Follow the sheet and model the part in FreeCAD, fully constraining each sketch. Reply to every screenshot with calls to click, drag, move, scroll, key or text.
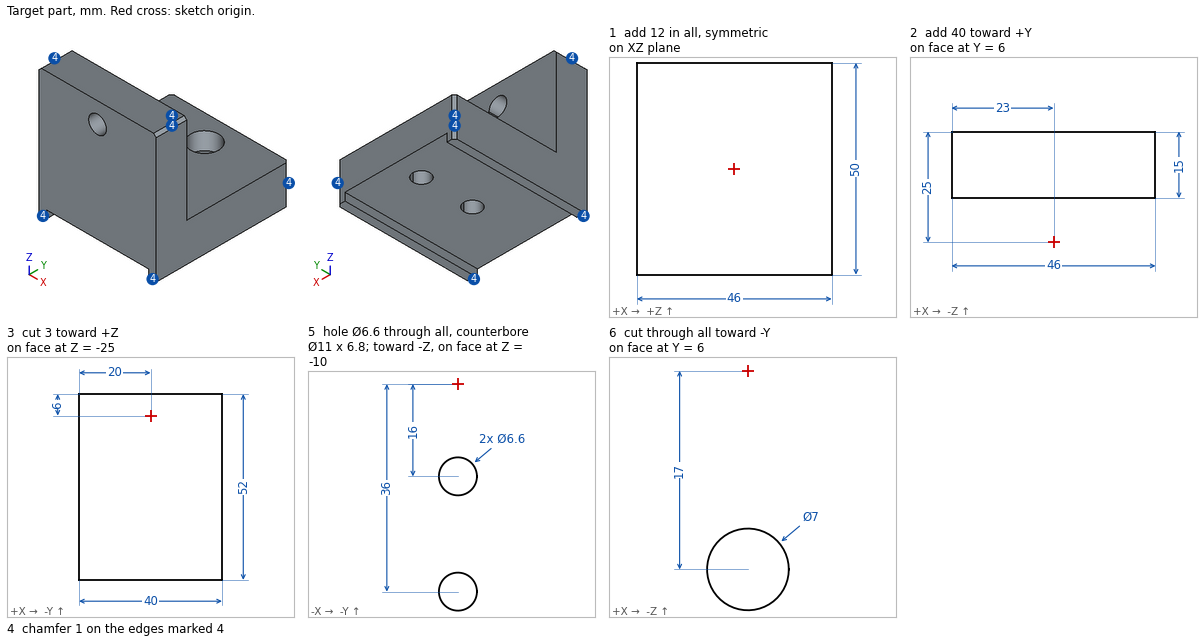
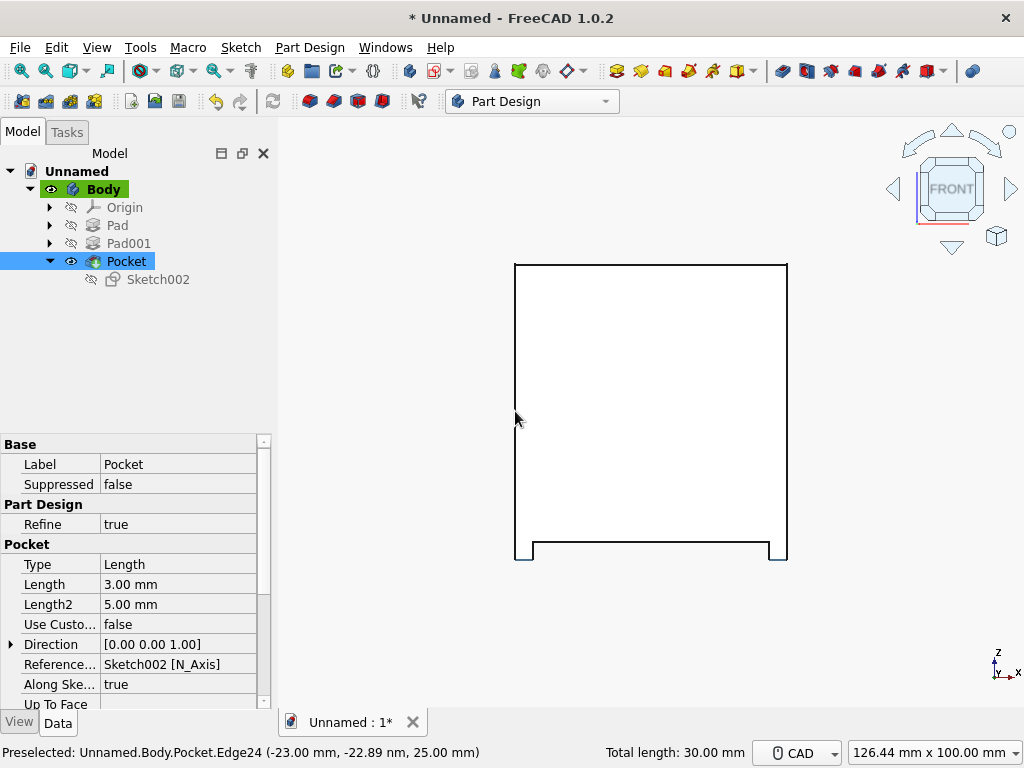
key(3)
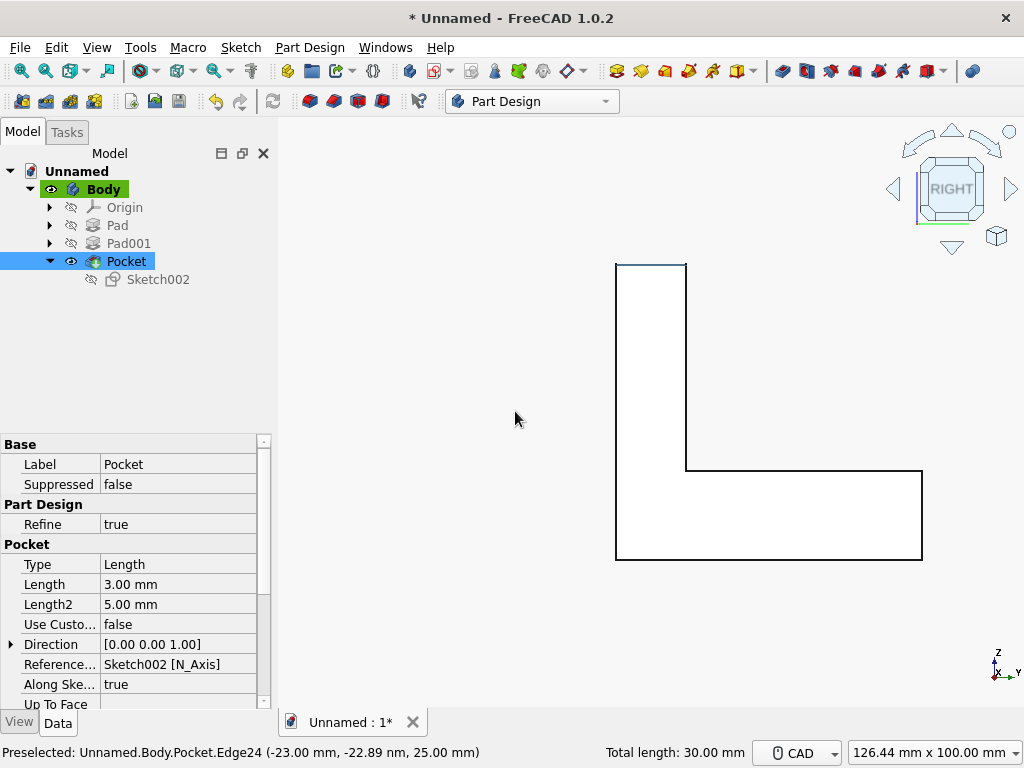
click(922, 514, ctrl)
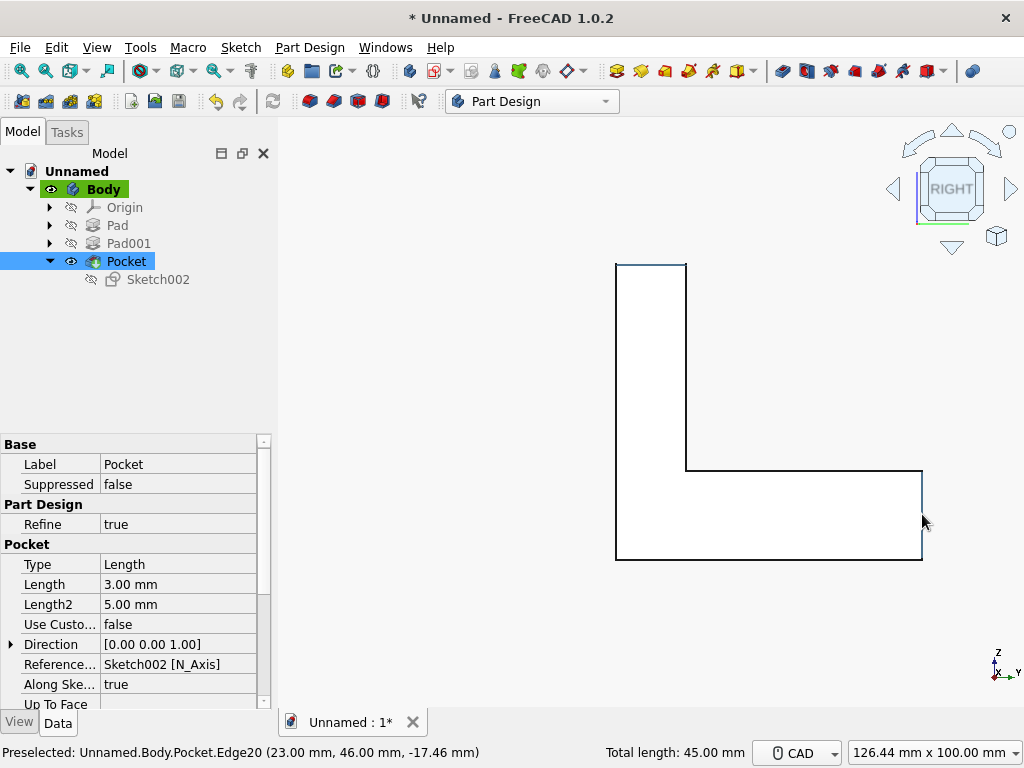
key(5)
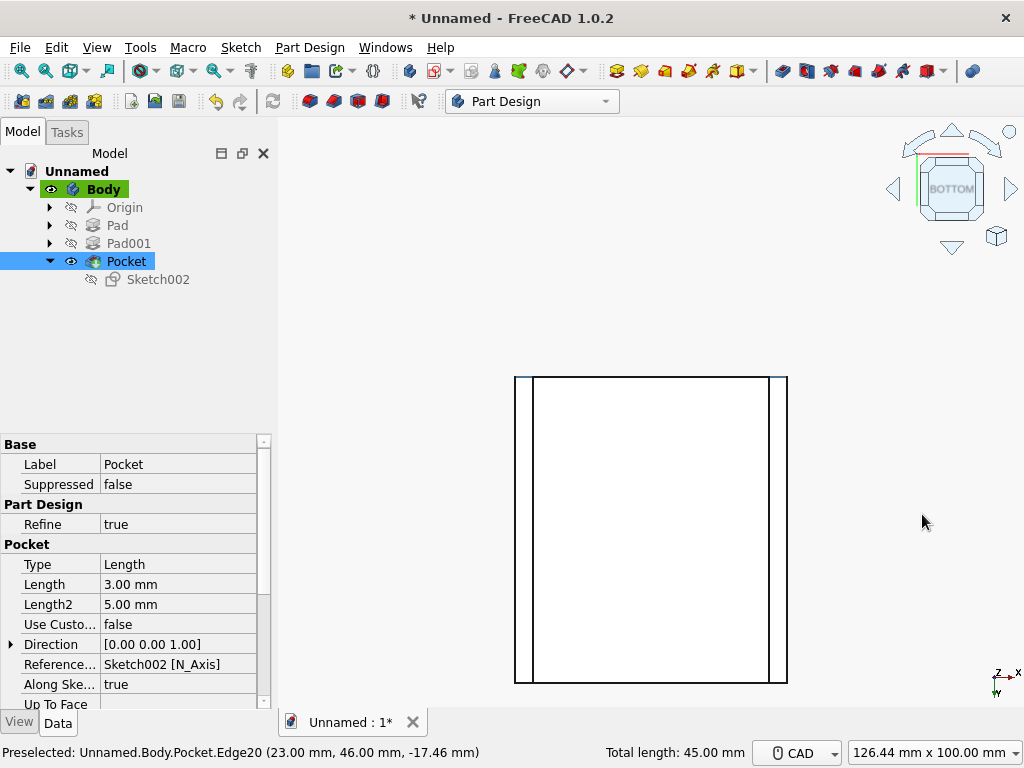
key(4)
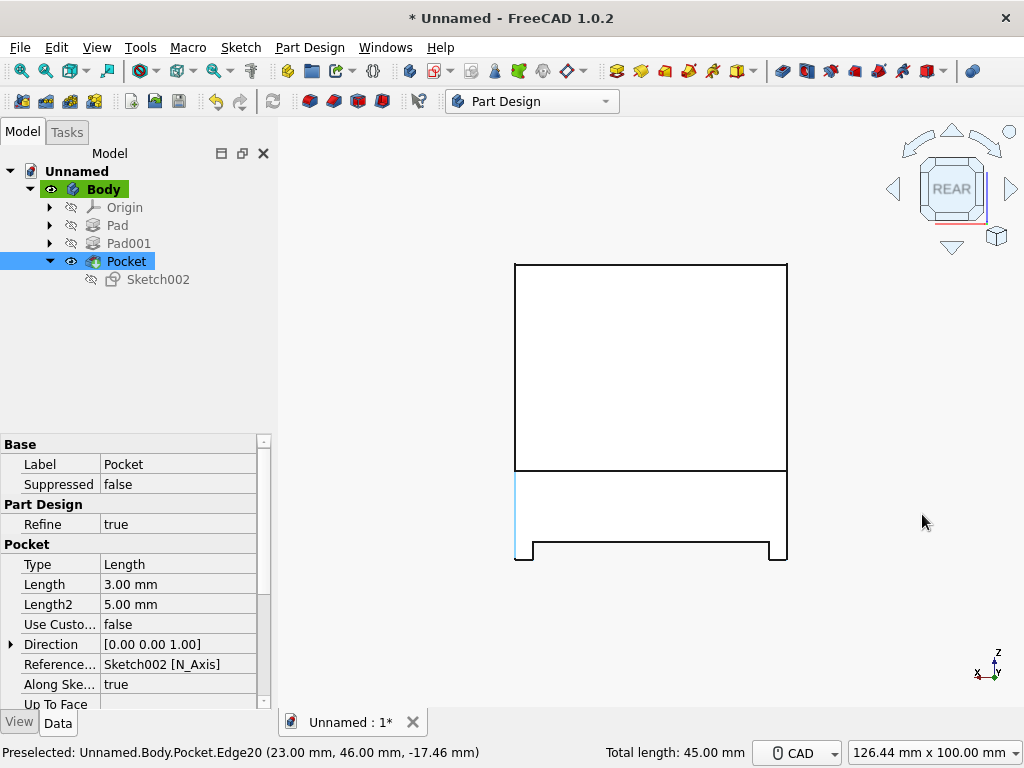
click(787, 514, ctrl)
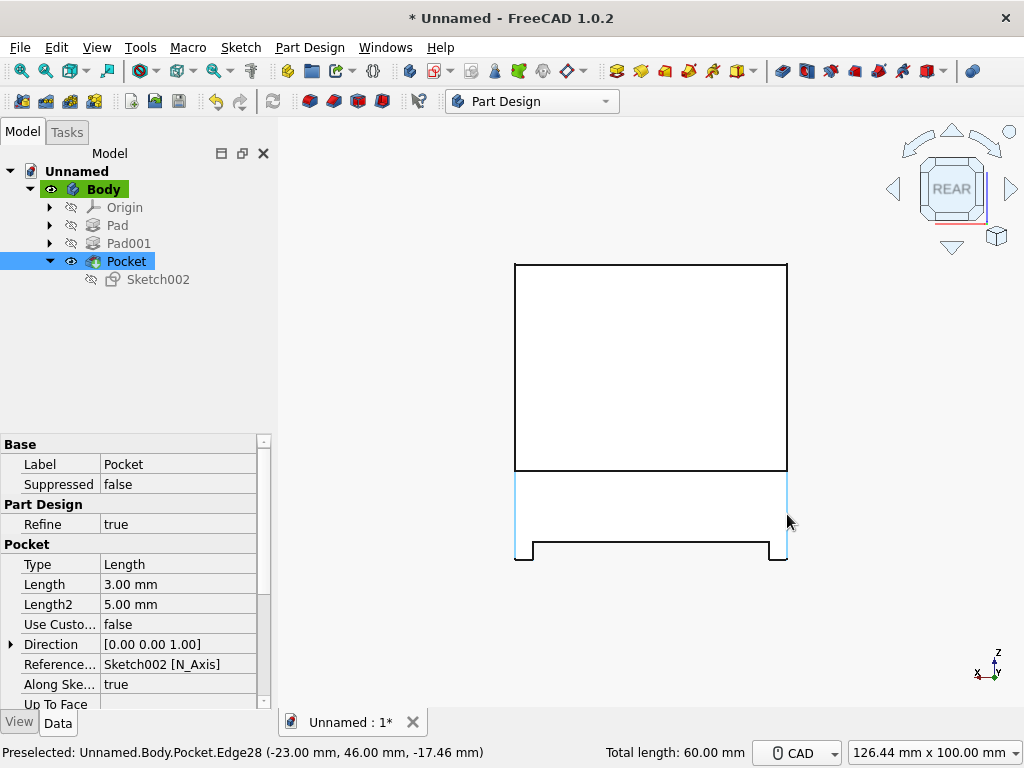
click(334, 102)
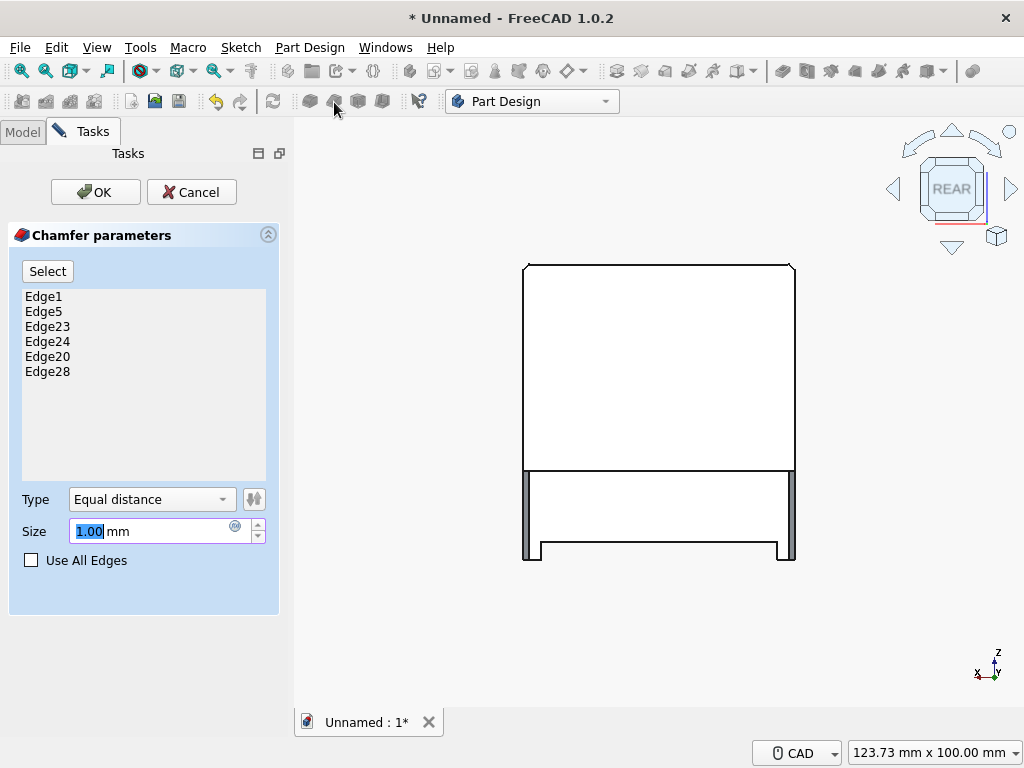
text(1)
key(Tab)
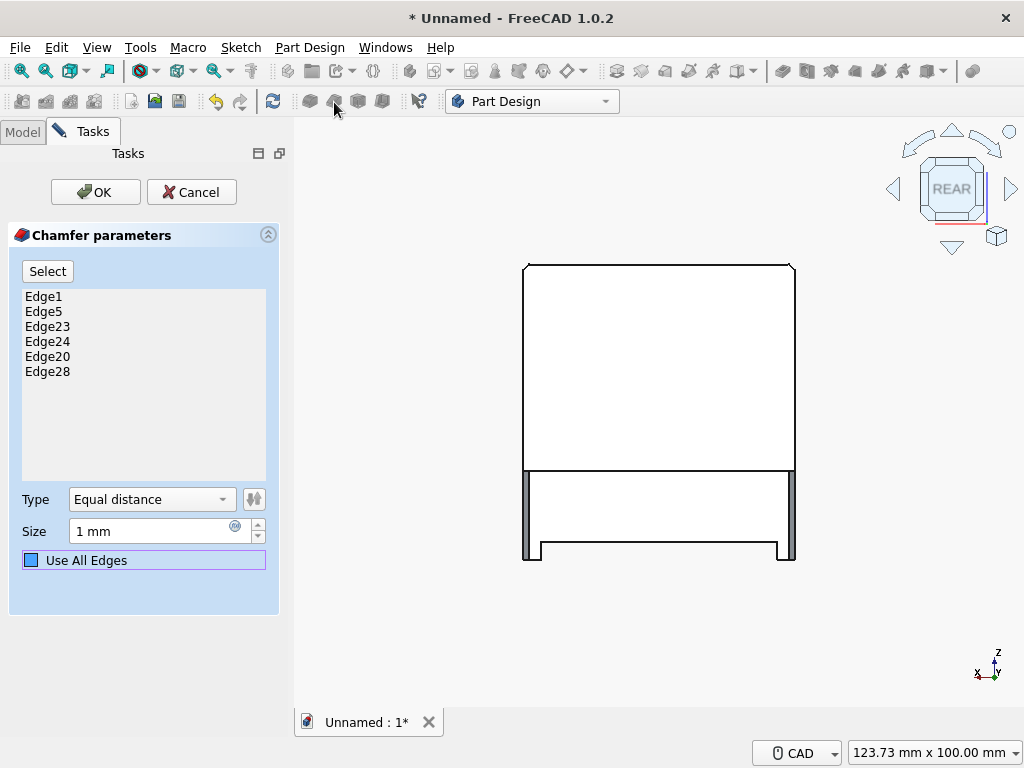
click(96, 192)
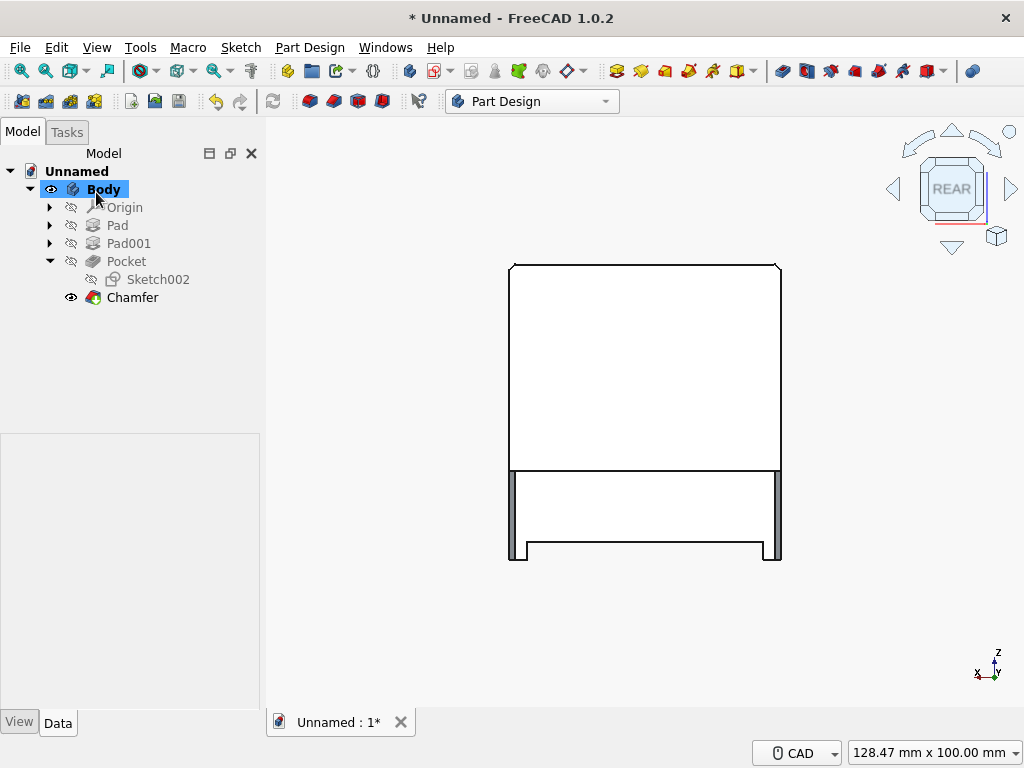
key(0)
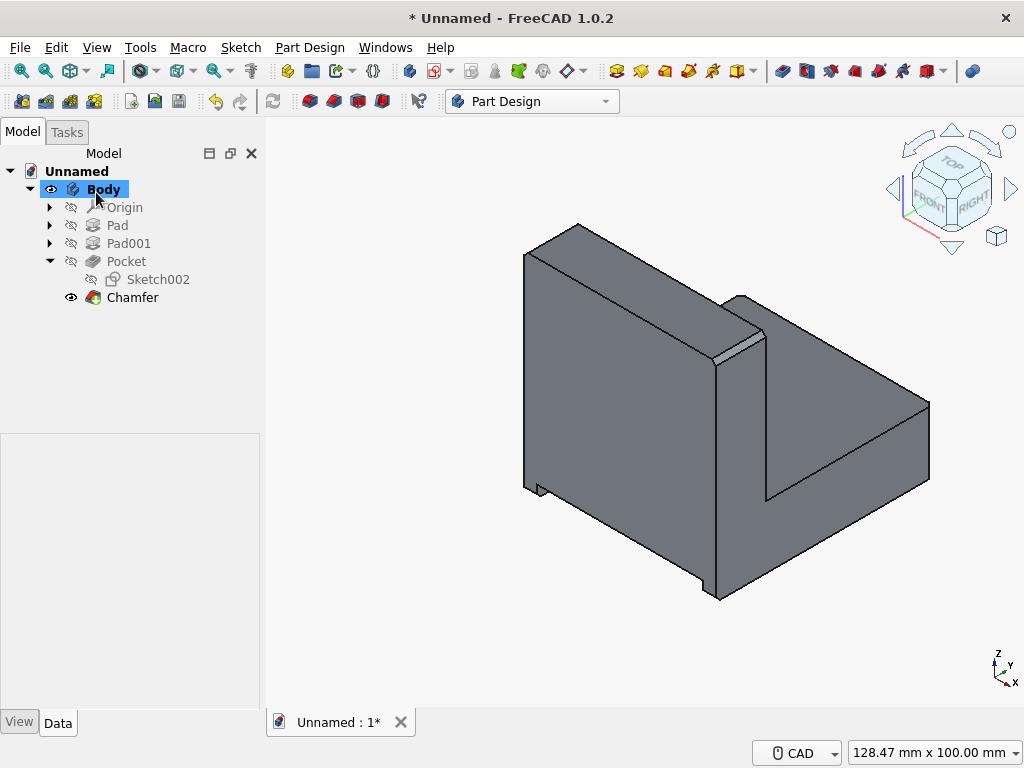
click(781, 412)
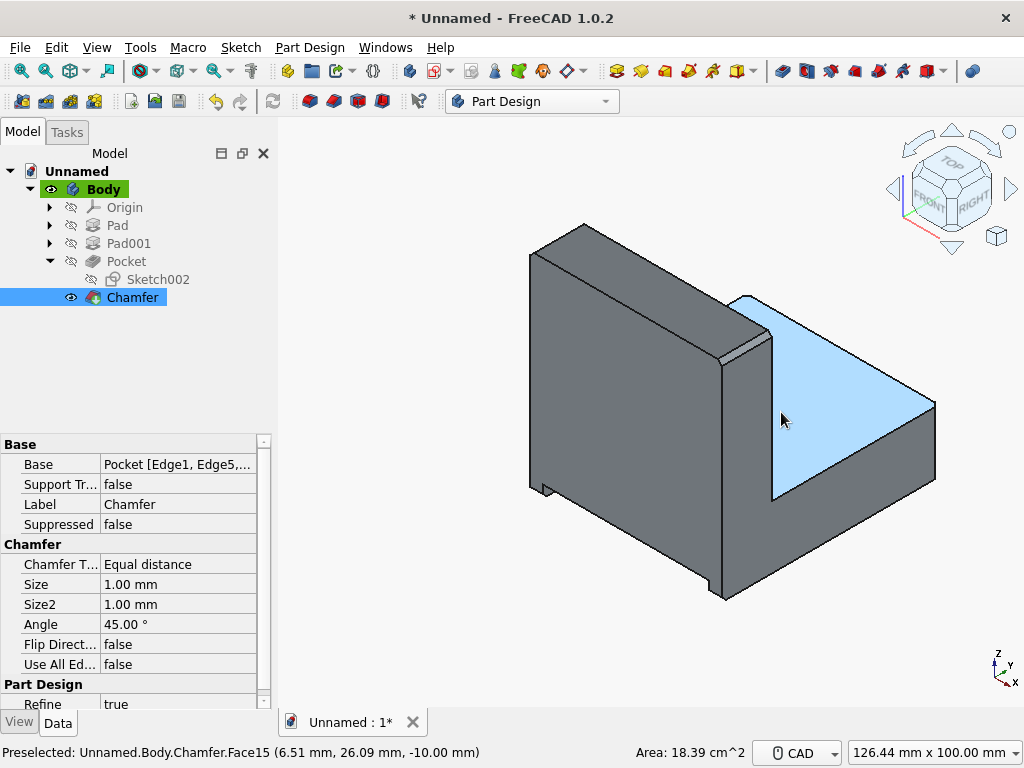
click(434, 72)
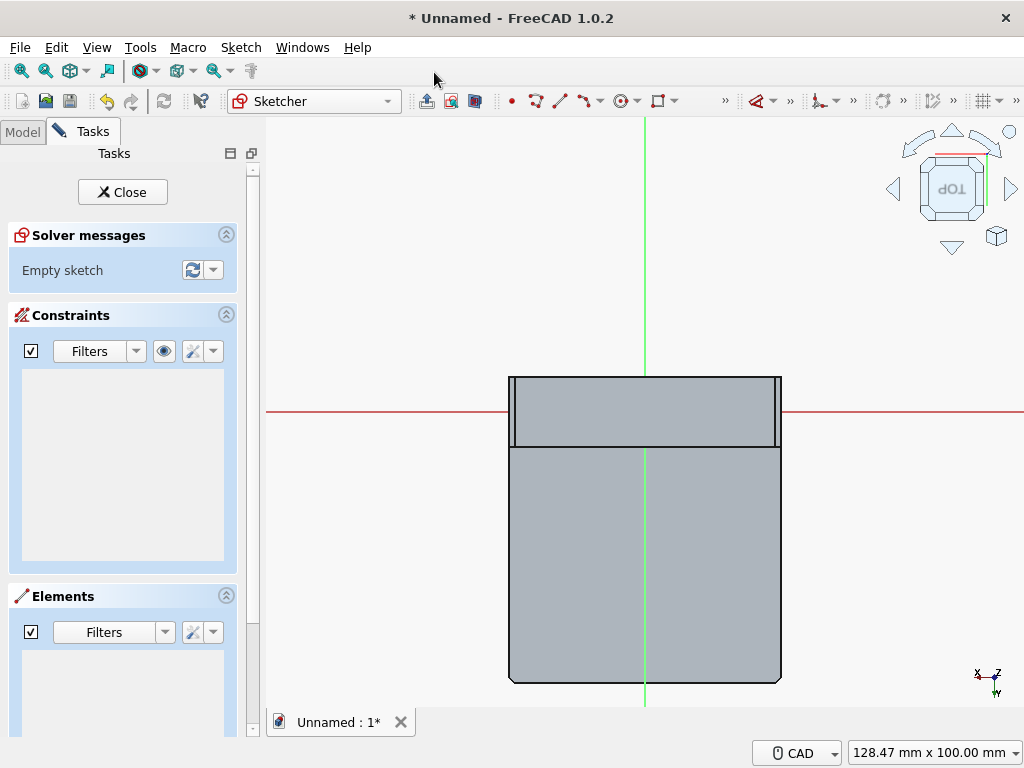
click(476, 102)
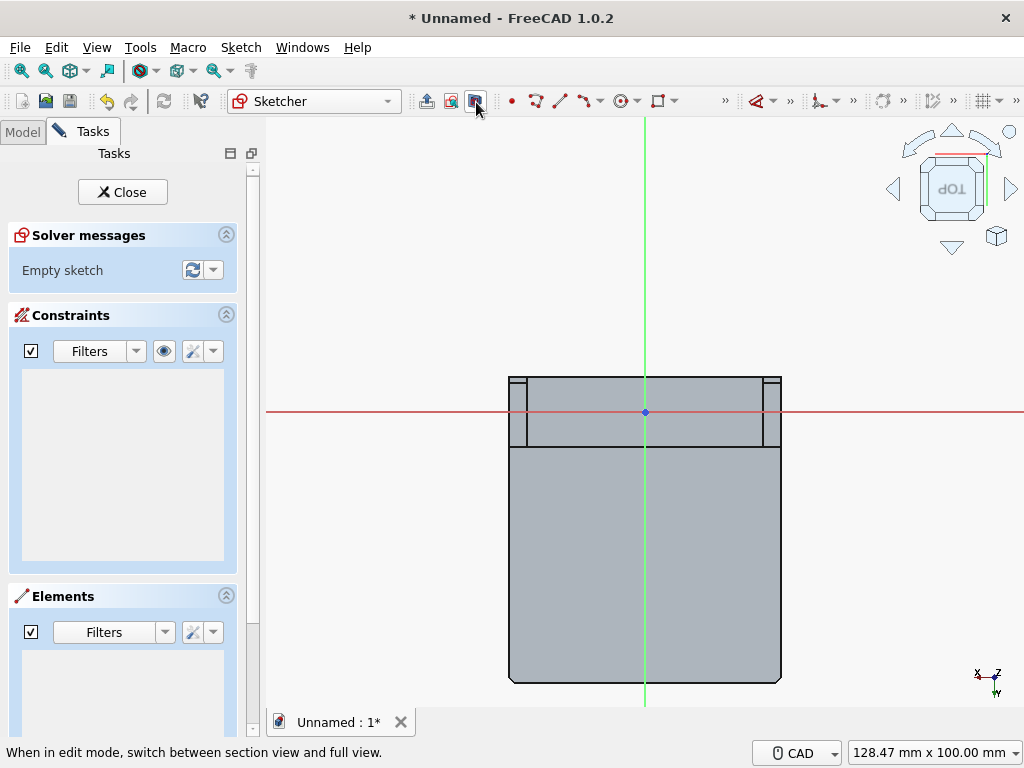
scroll(784, 679, up, 2)